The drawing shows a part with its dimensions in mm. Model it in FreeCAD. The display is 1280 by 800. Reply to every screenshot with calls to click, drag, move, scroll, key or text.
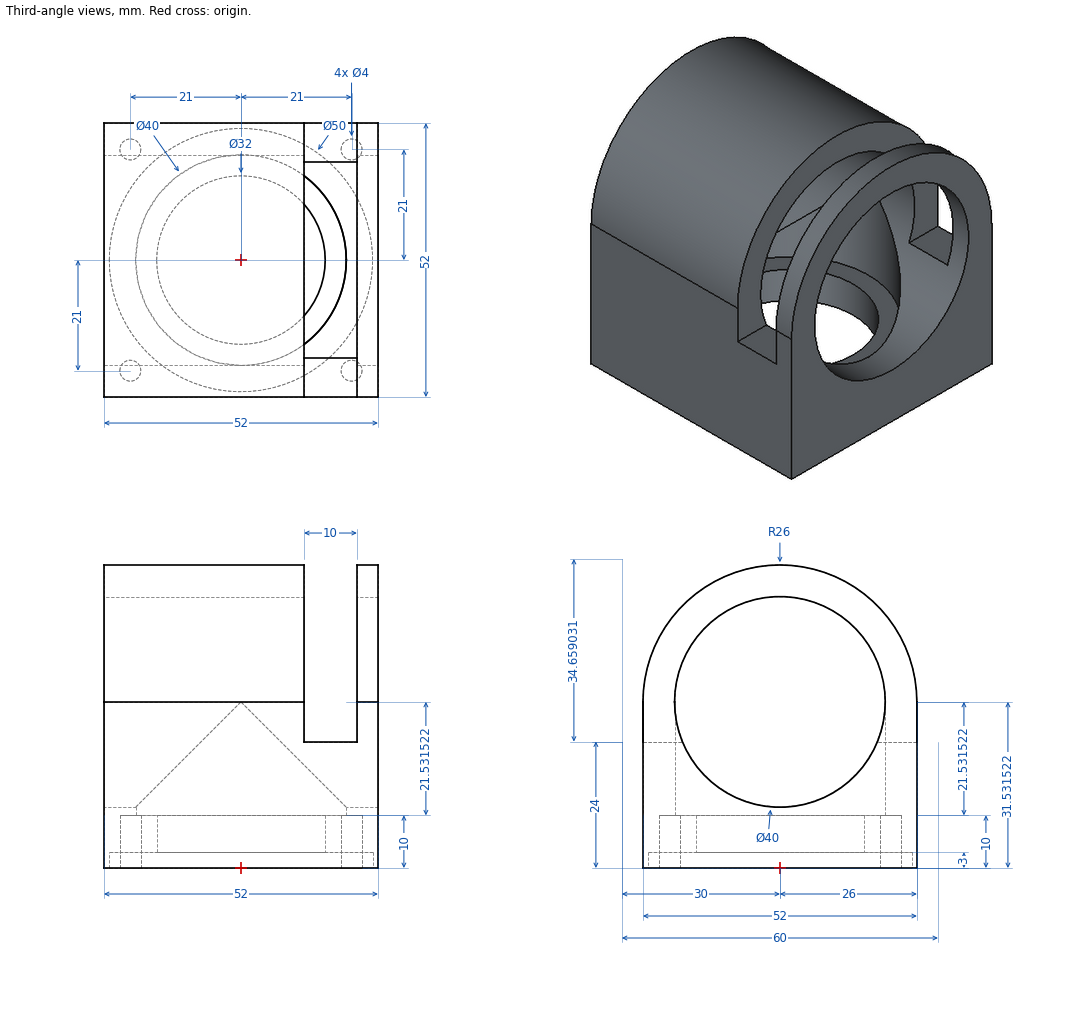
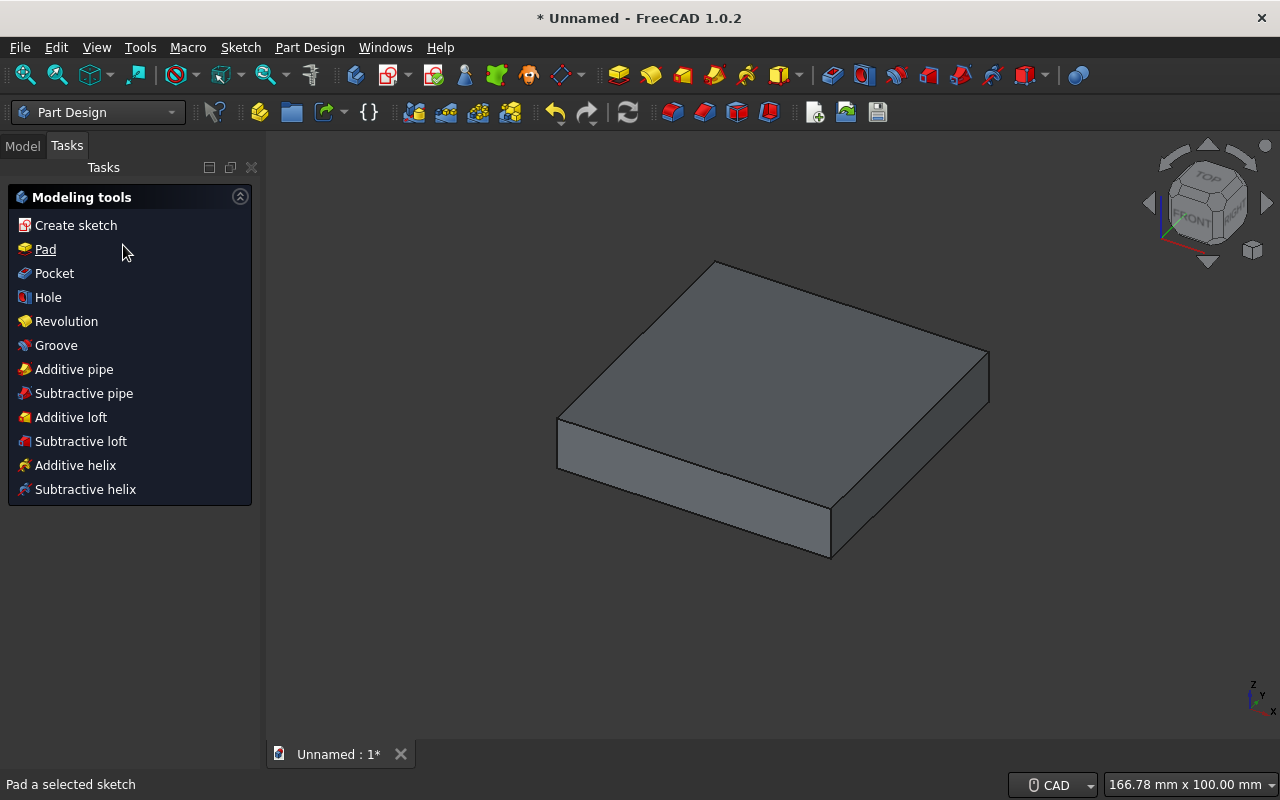
click(834, 76)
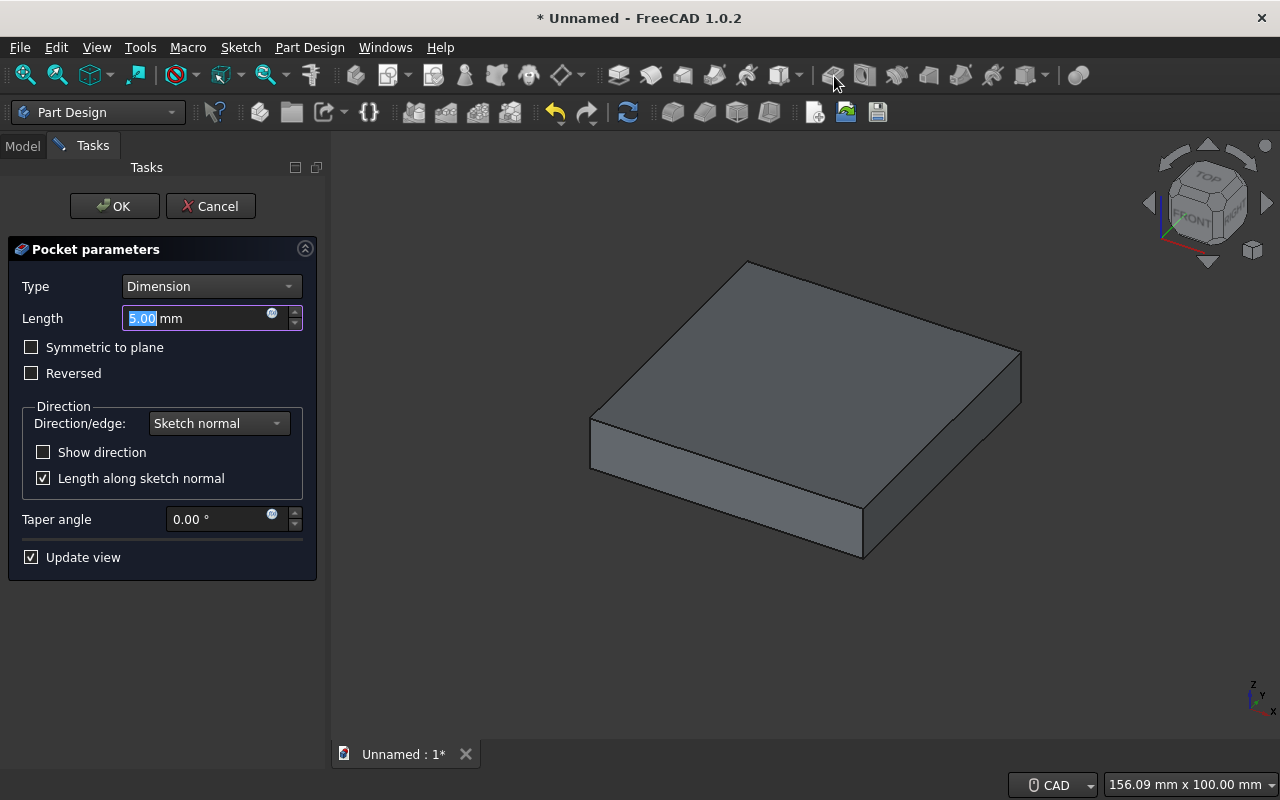
text(10)
key(Tab)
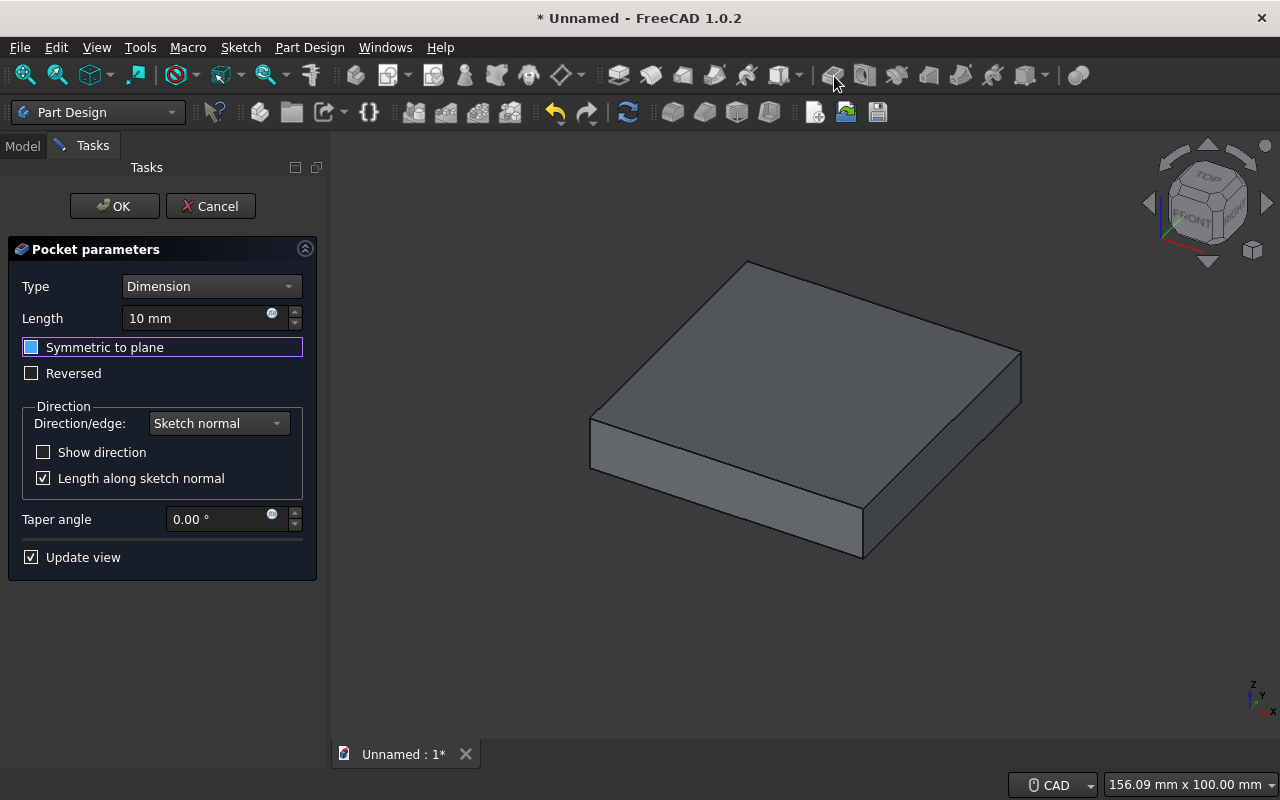
click(30, 373)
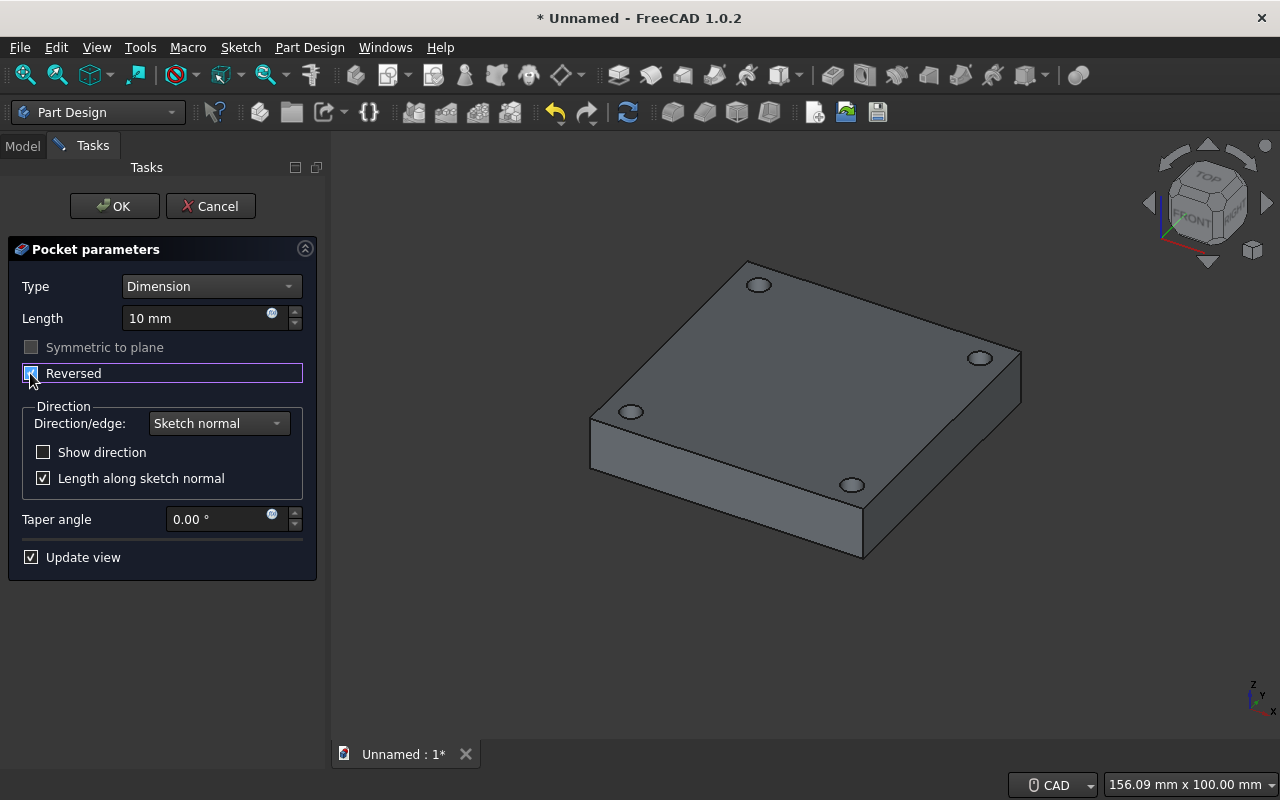
click(115, 206)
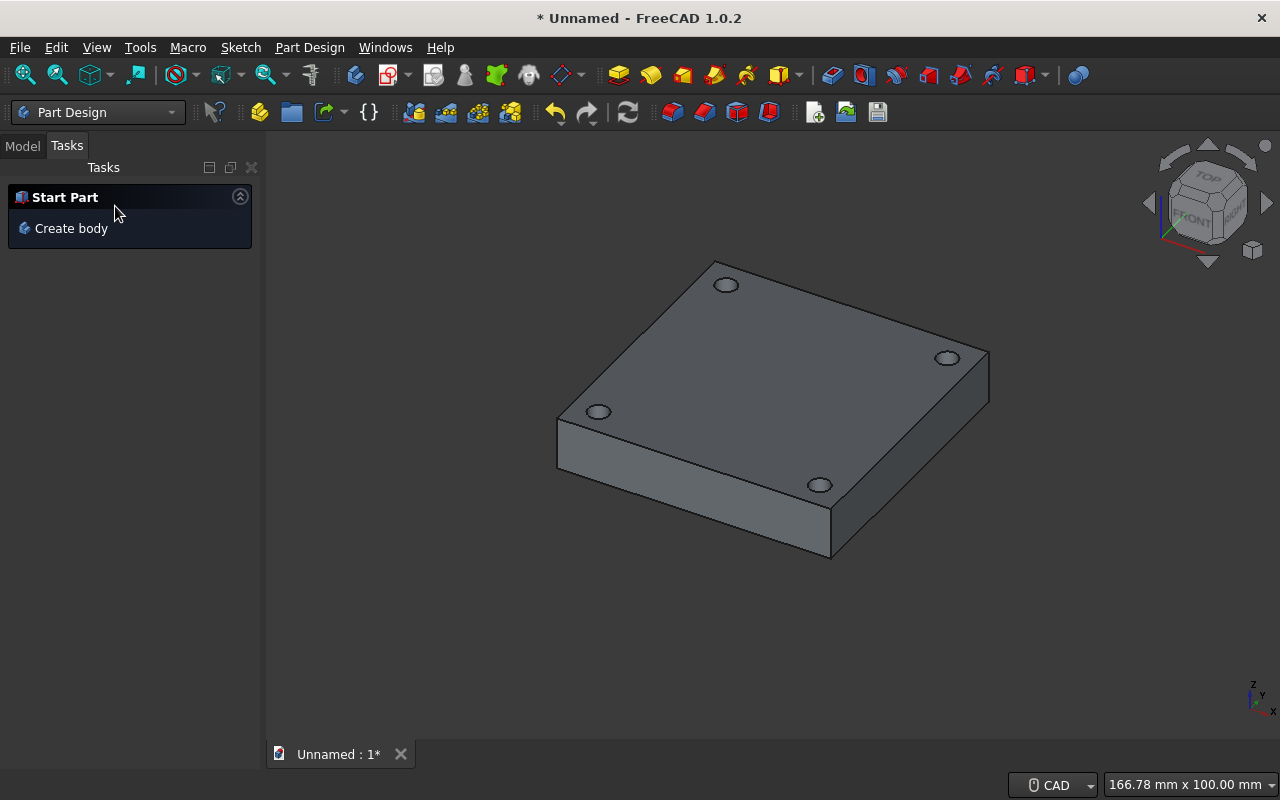
click(388, 76)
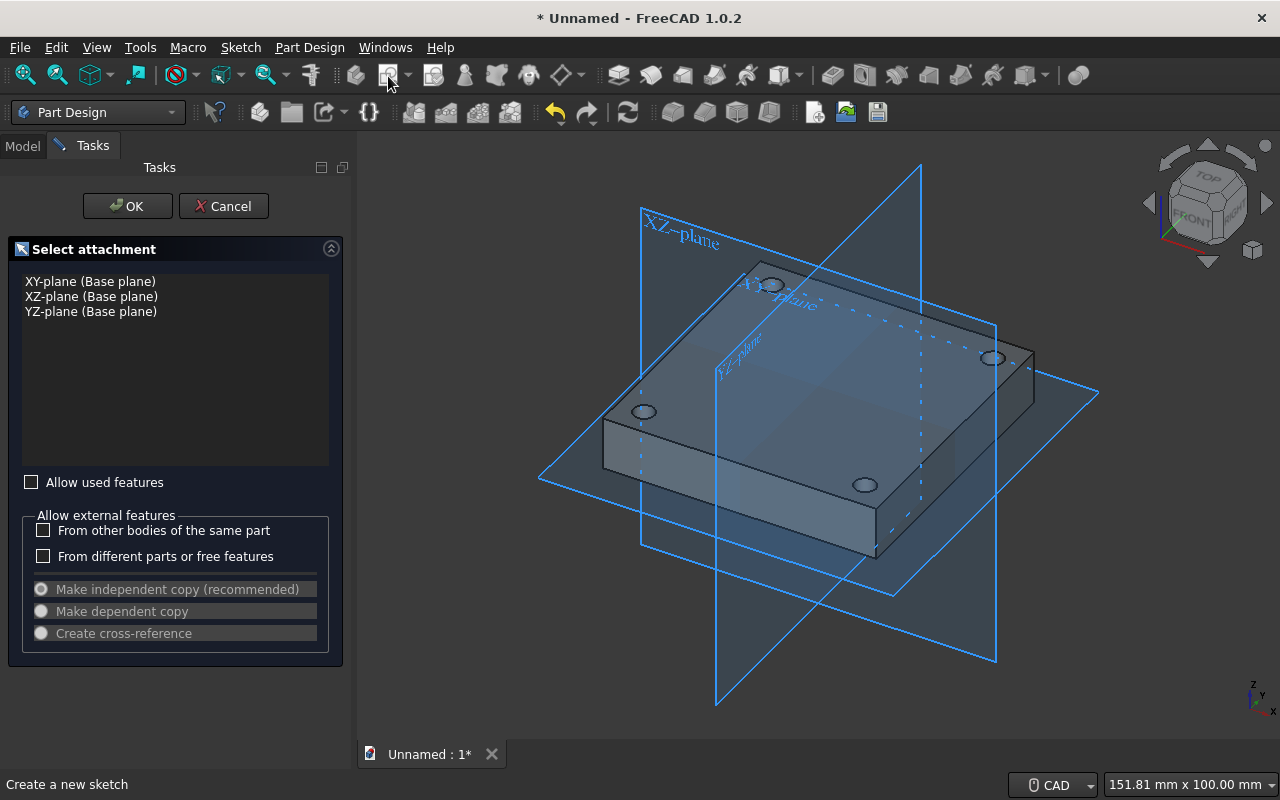
click(82, 282)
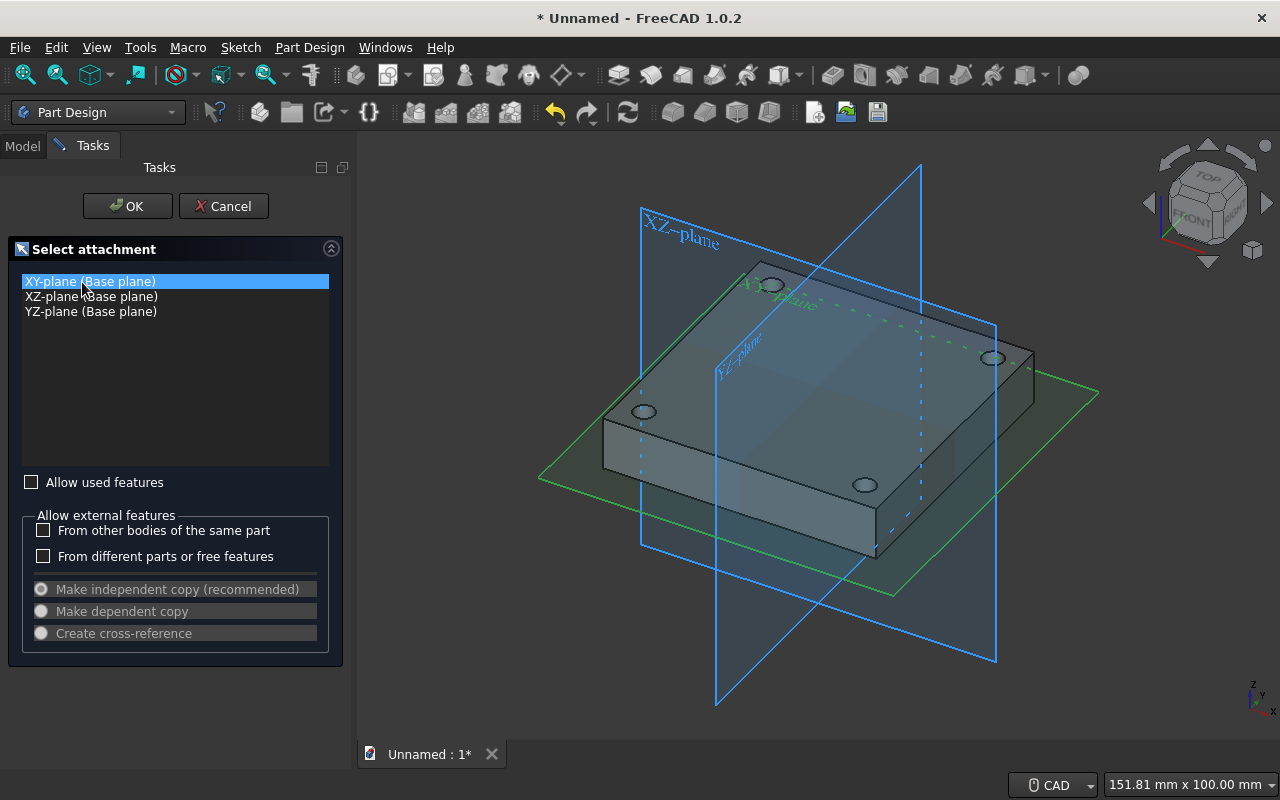
click(128, 206)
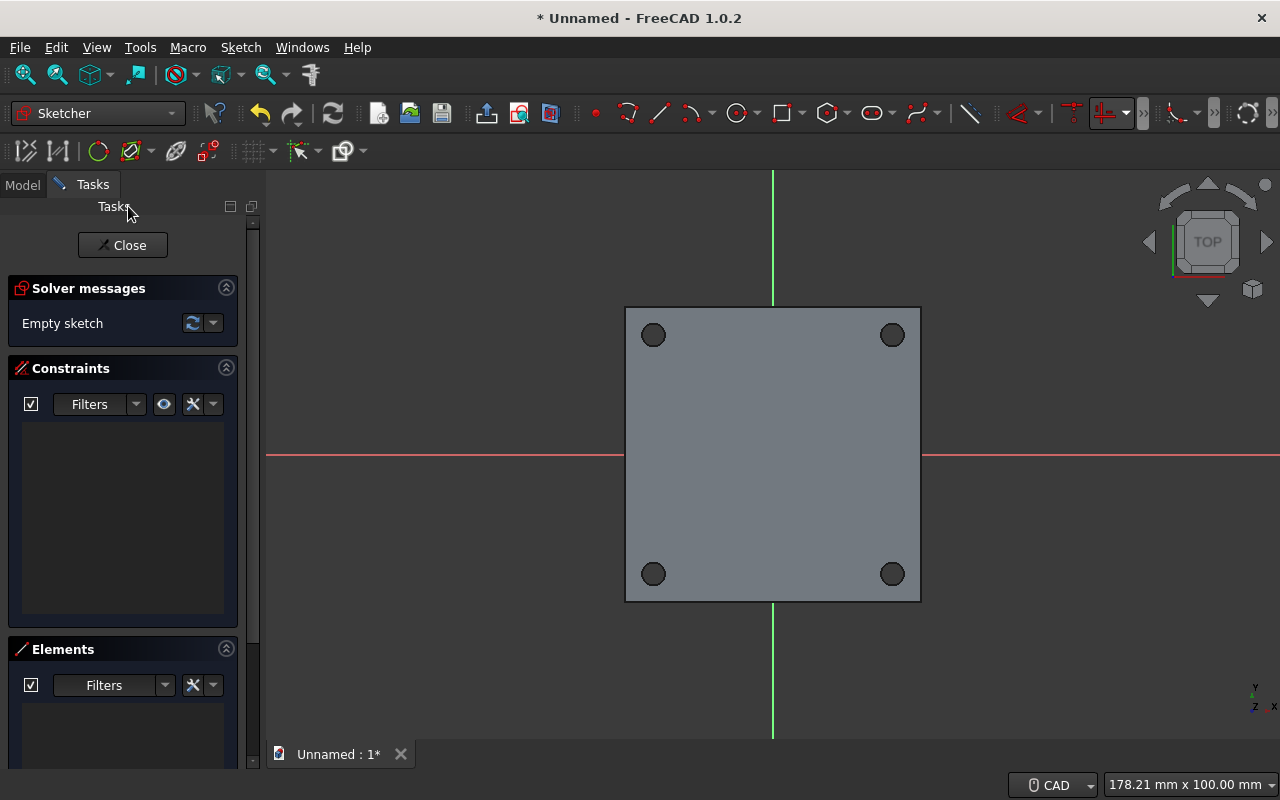
click(552, 114)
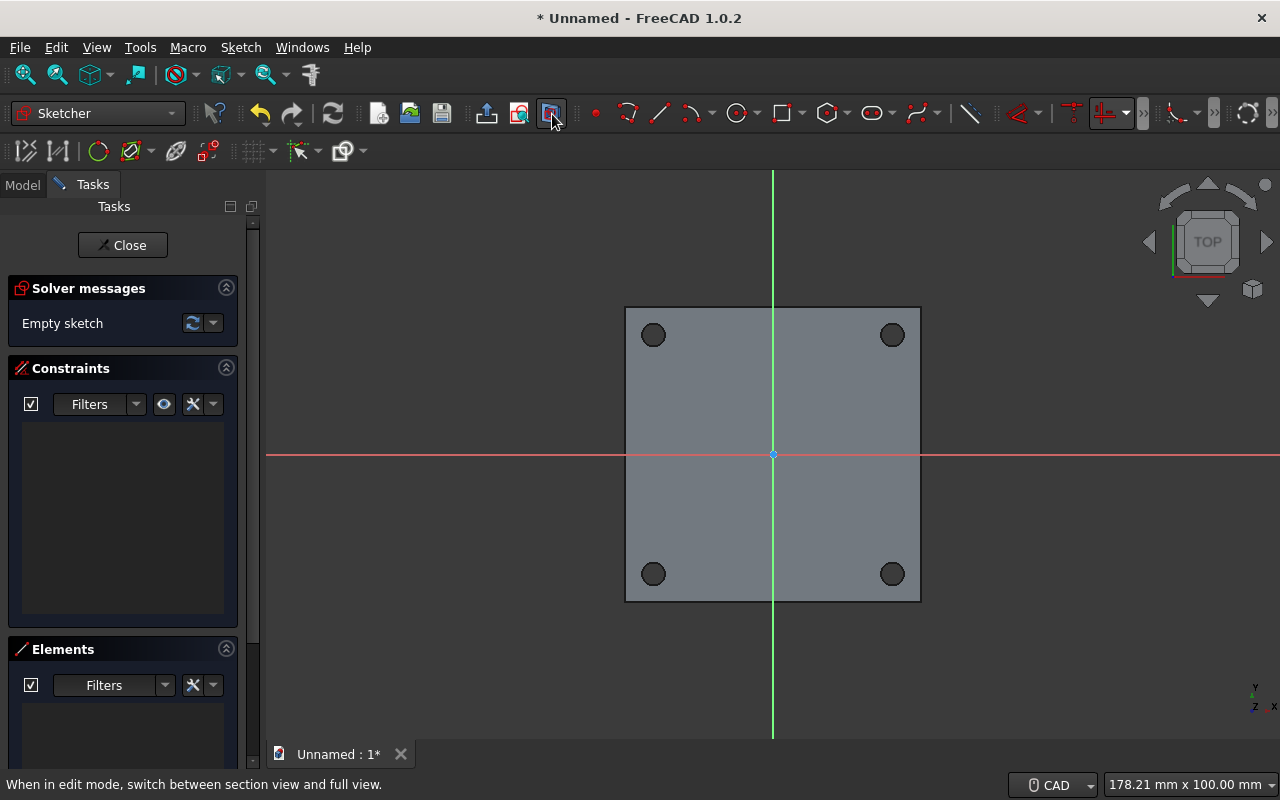
click(738, 114)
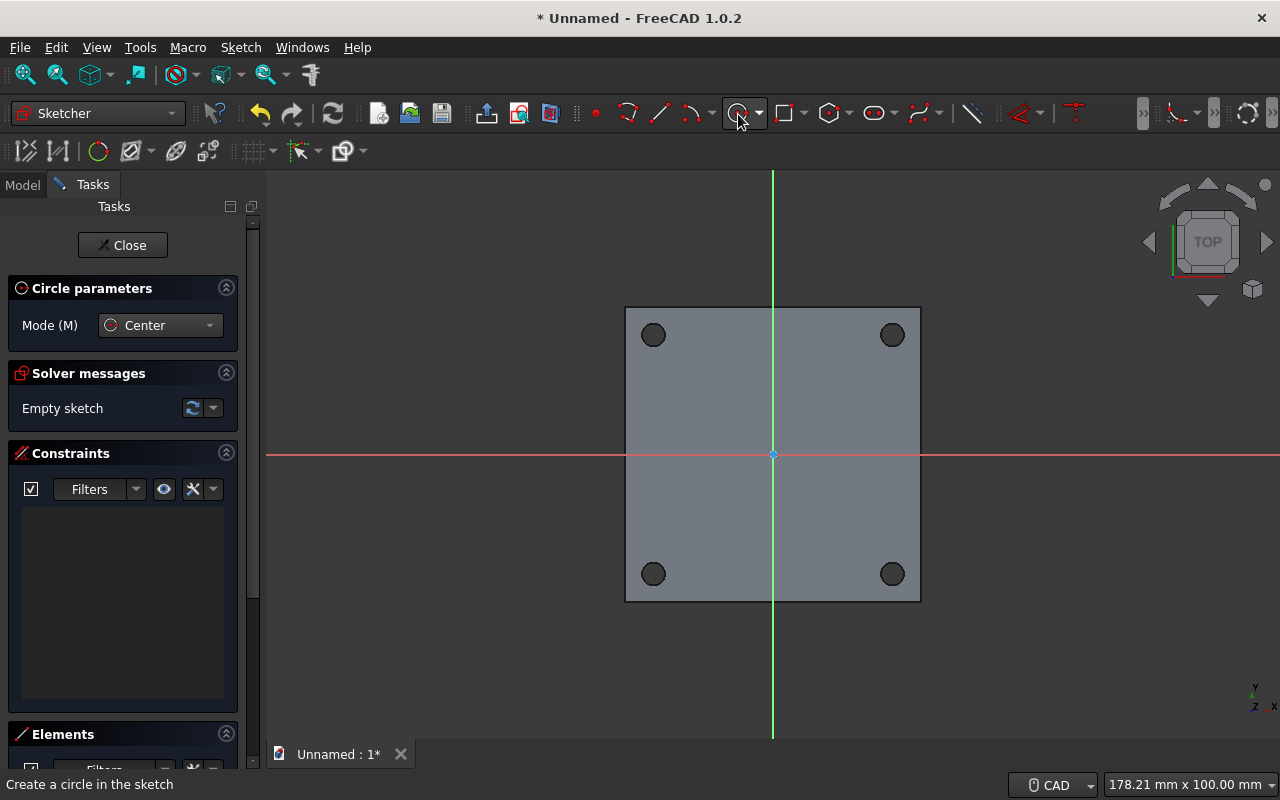
click(773, 454)
click(874, 354)
key(Escape)